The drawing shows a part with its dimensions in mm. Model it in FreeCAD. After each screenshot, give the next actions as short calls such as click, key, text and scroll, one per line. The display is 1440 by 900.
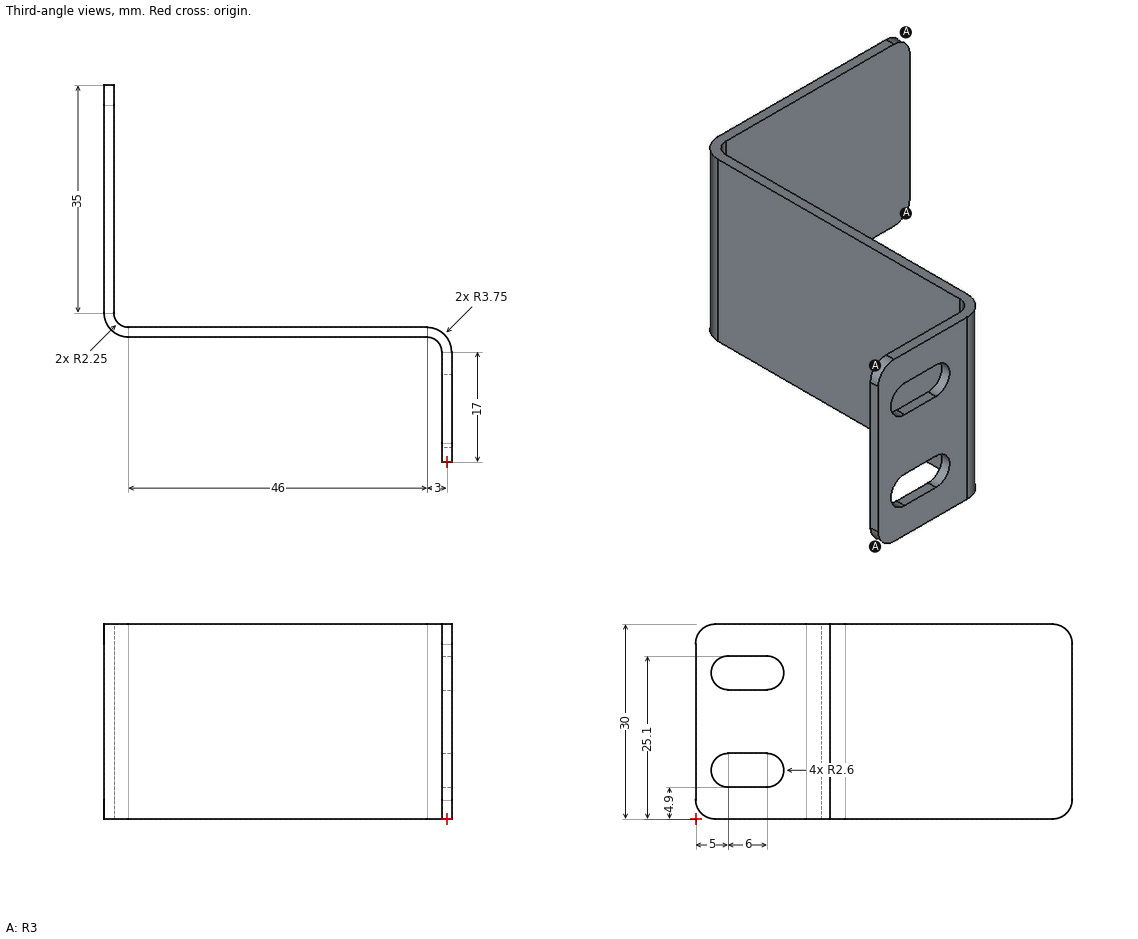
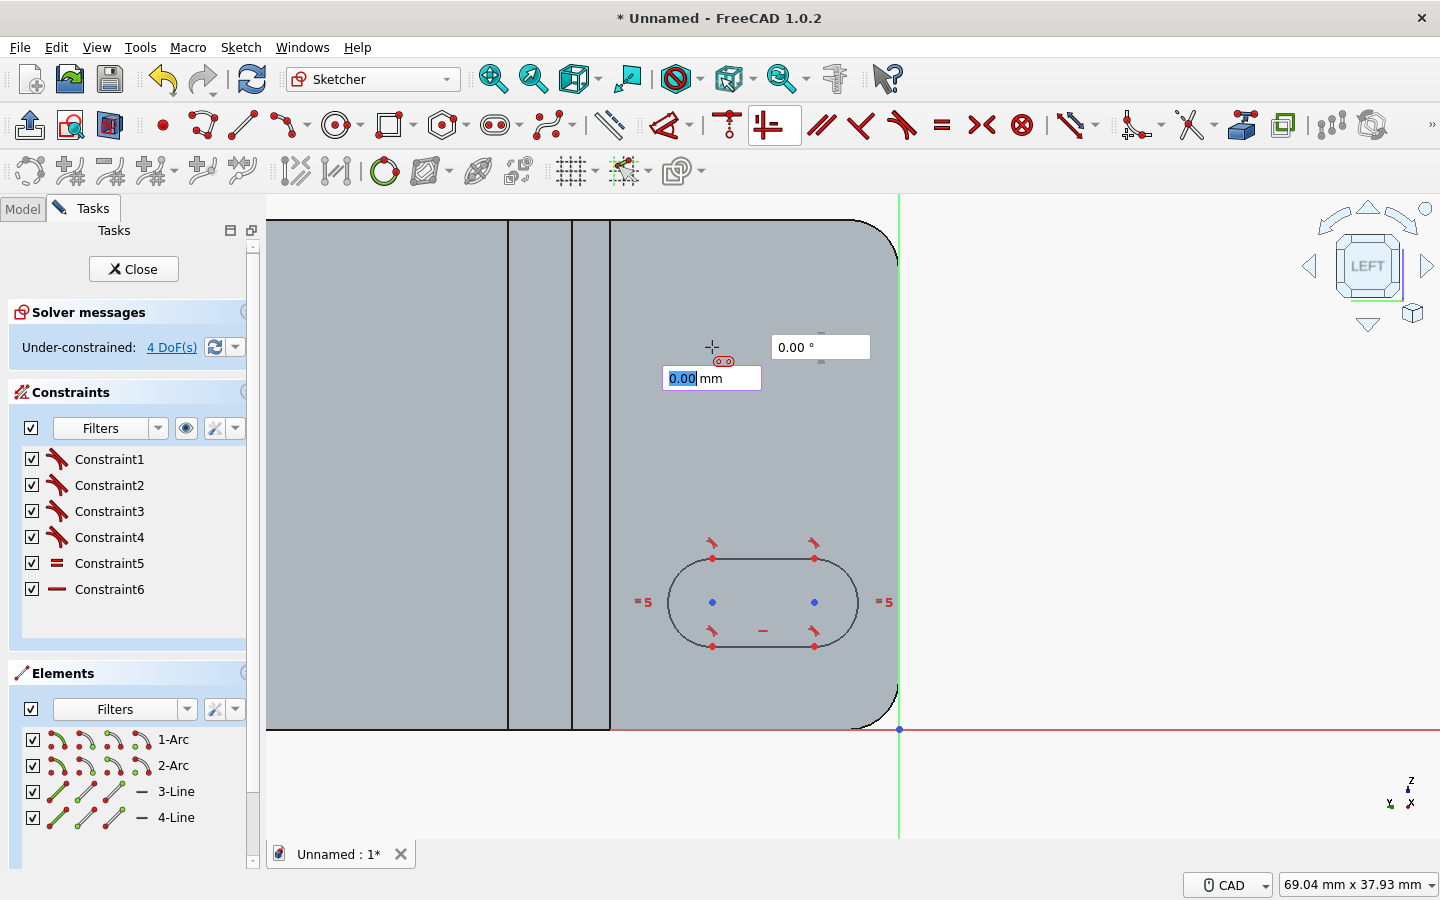
click(814, 347)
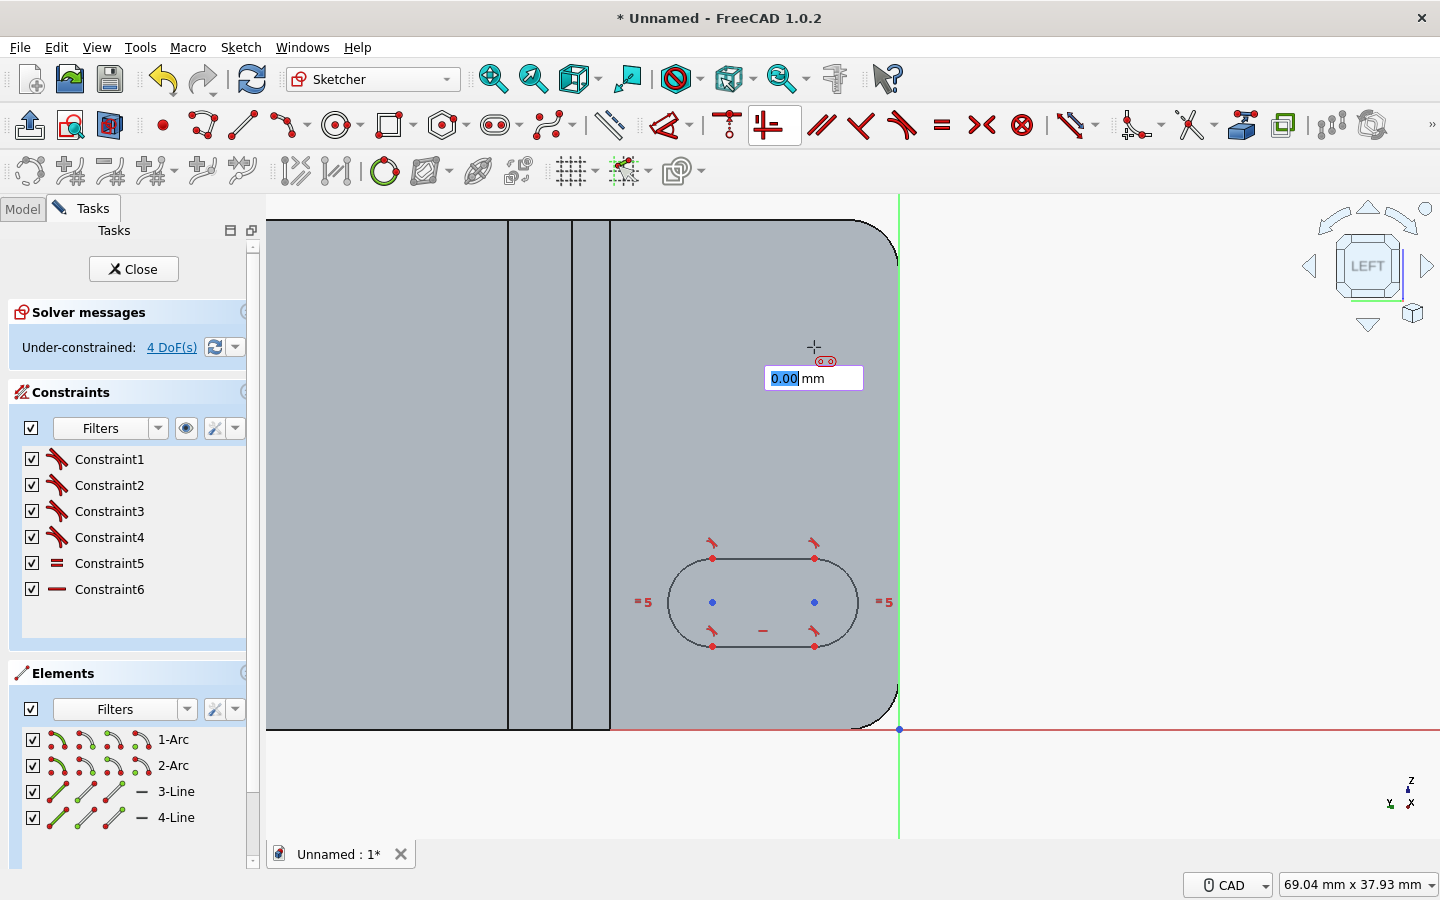
click(763, 303)
key(Escape)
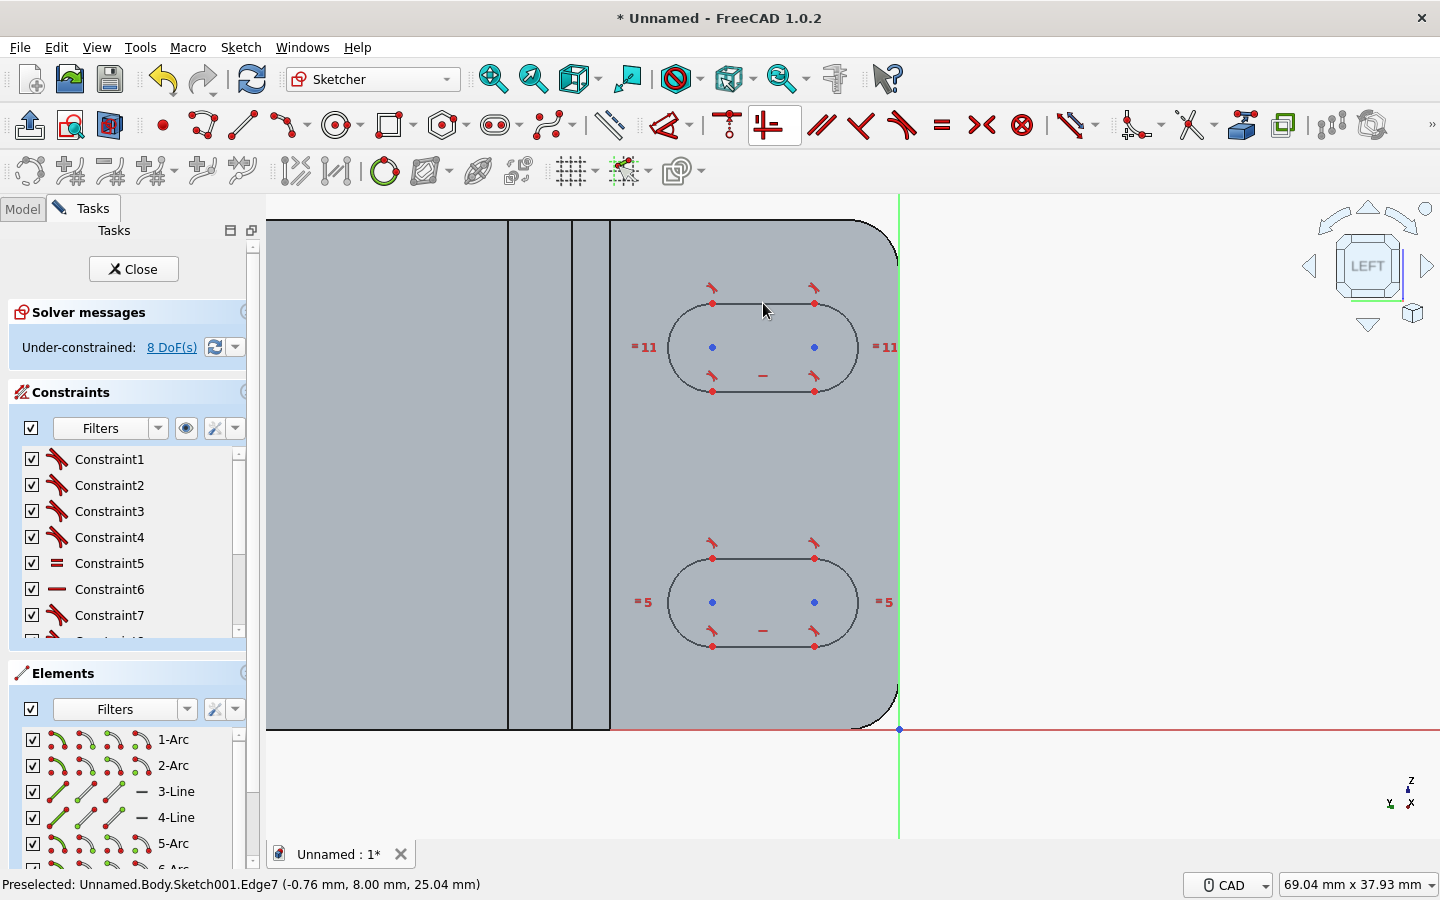
click(676, 577)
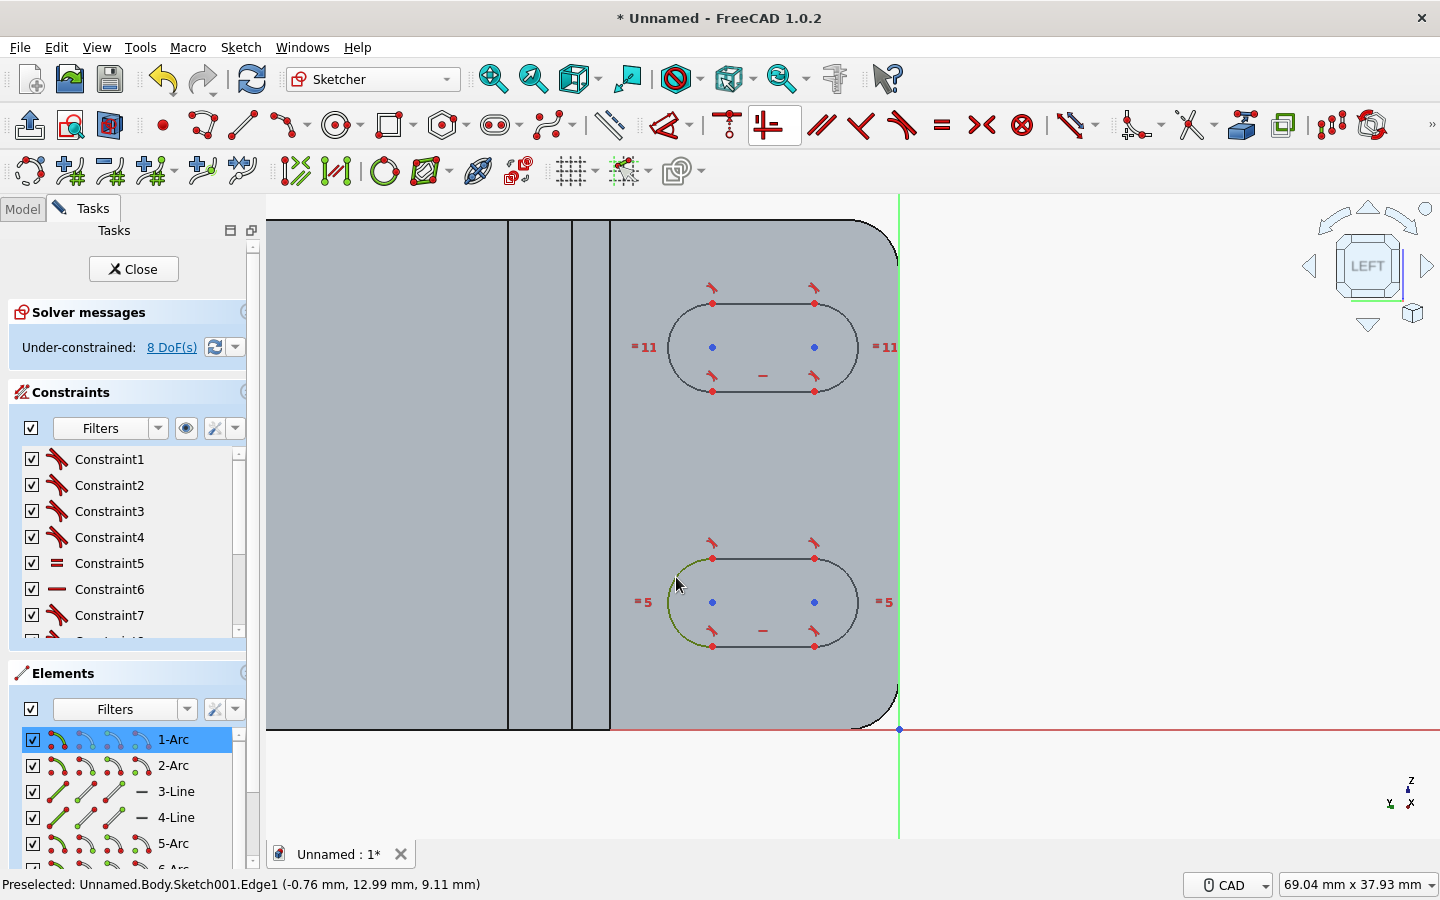
click(676, 322)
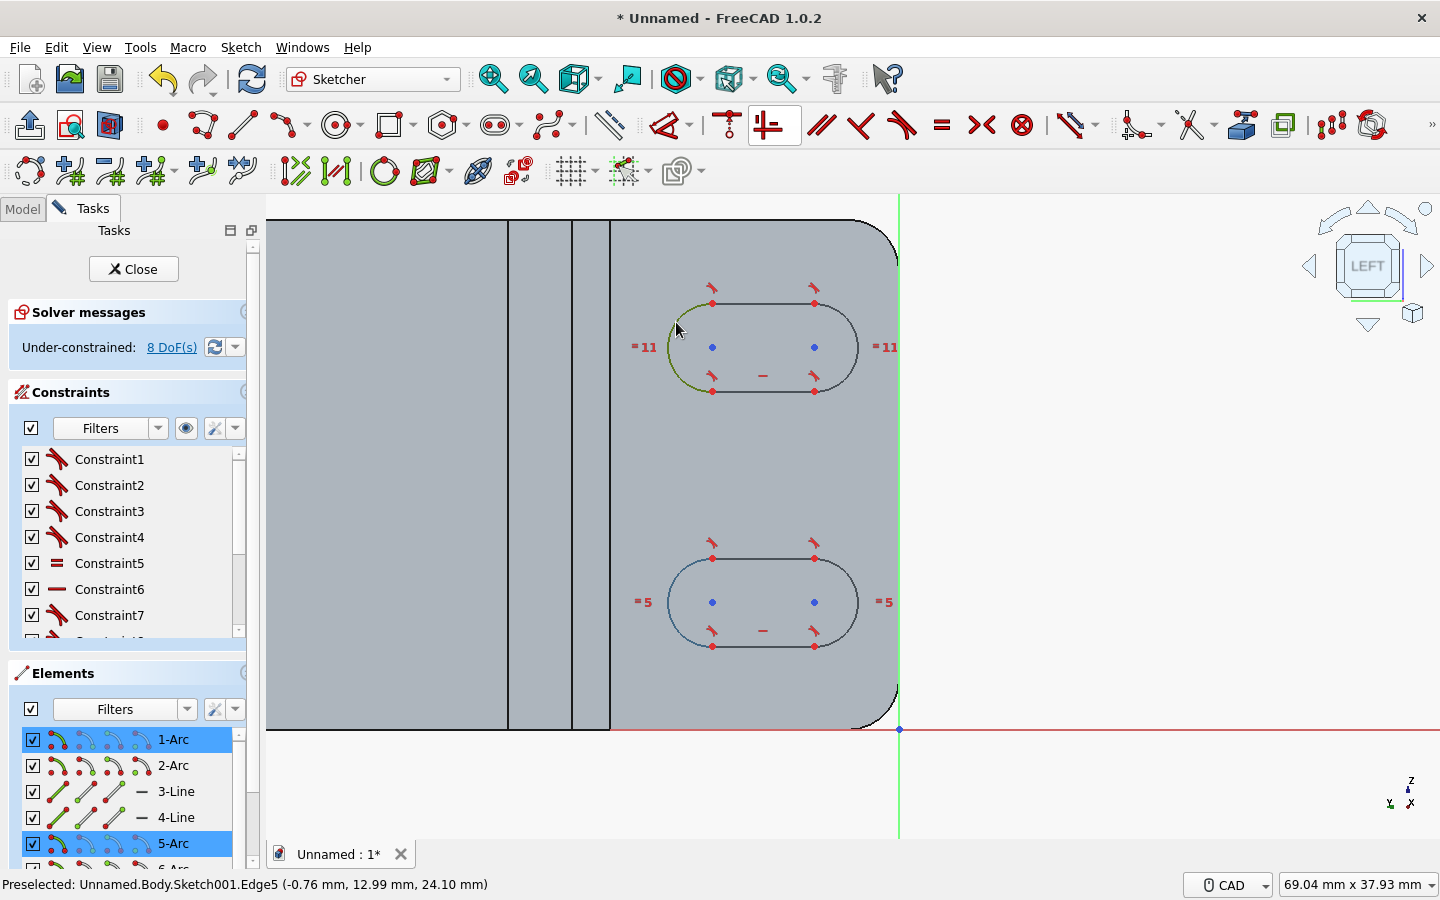
key(e)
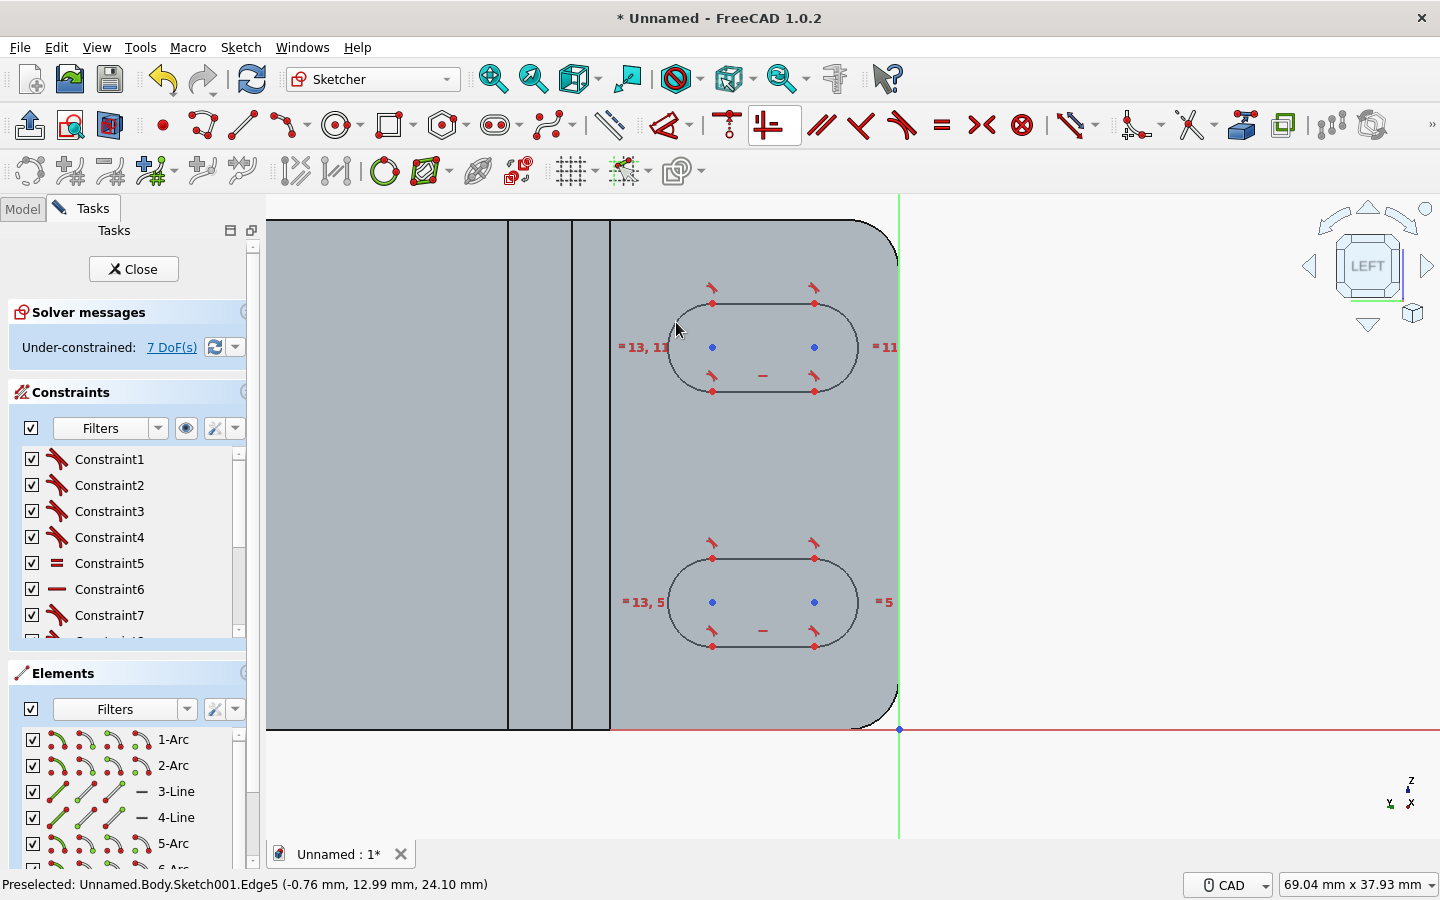
click(664, 126)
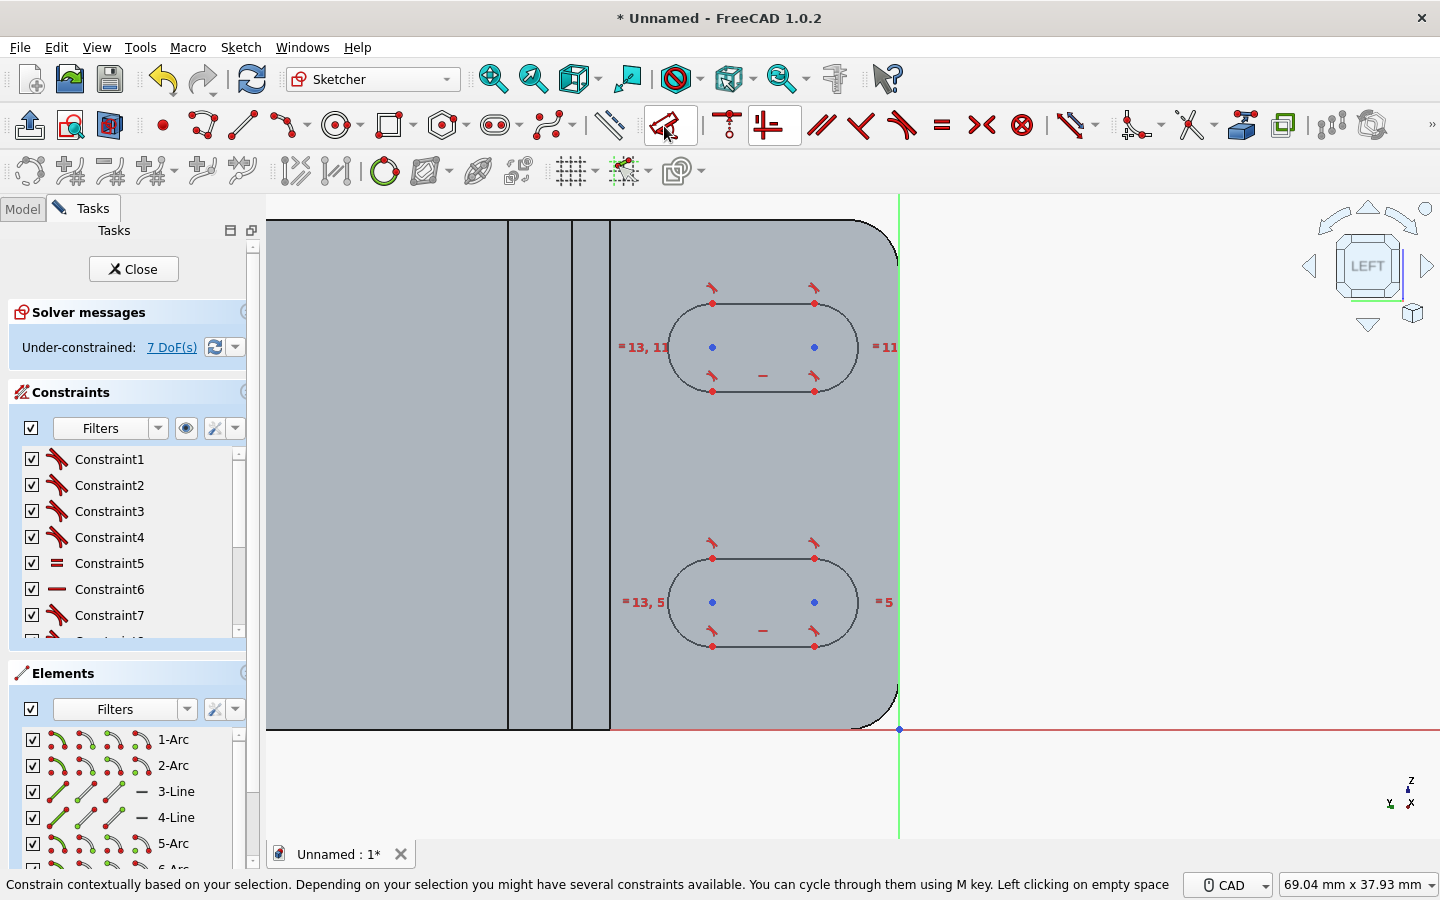
click(676, 577)
click(650, 558)